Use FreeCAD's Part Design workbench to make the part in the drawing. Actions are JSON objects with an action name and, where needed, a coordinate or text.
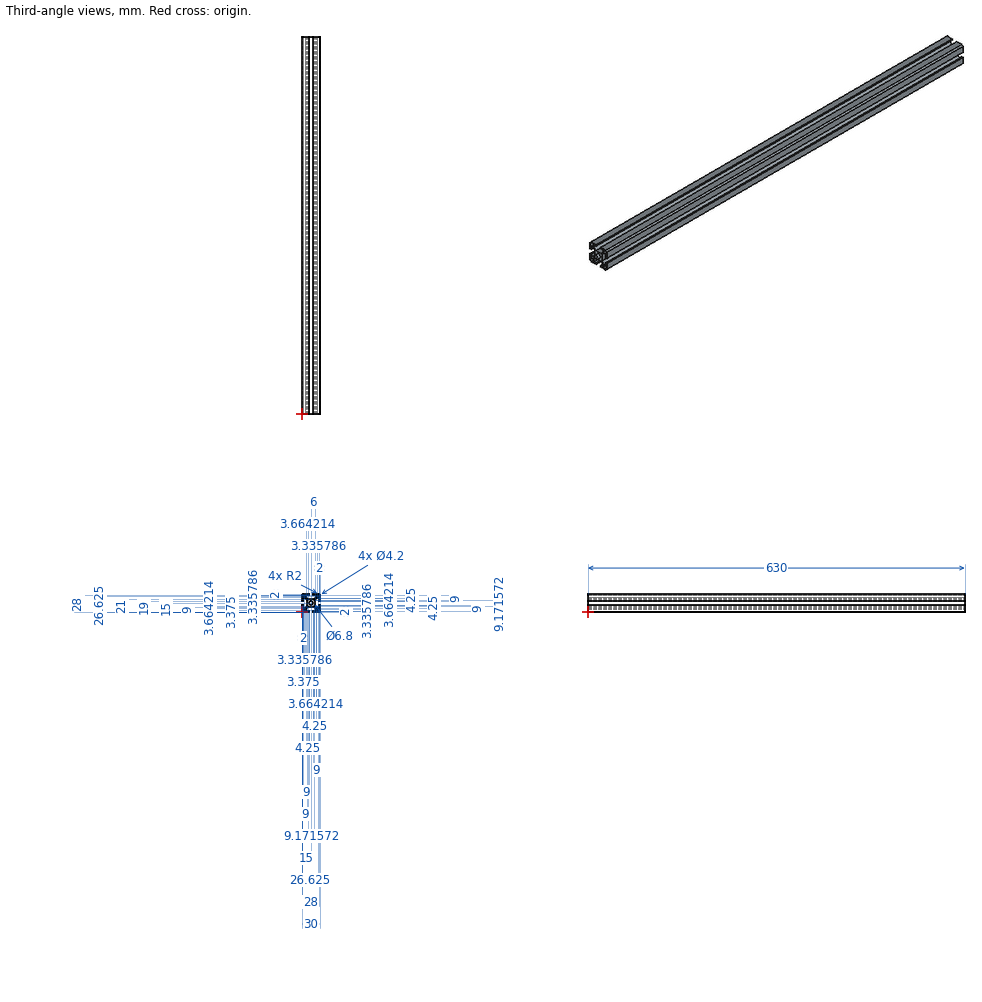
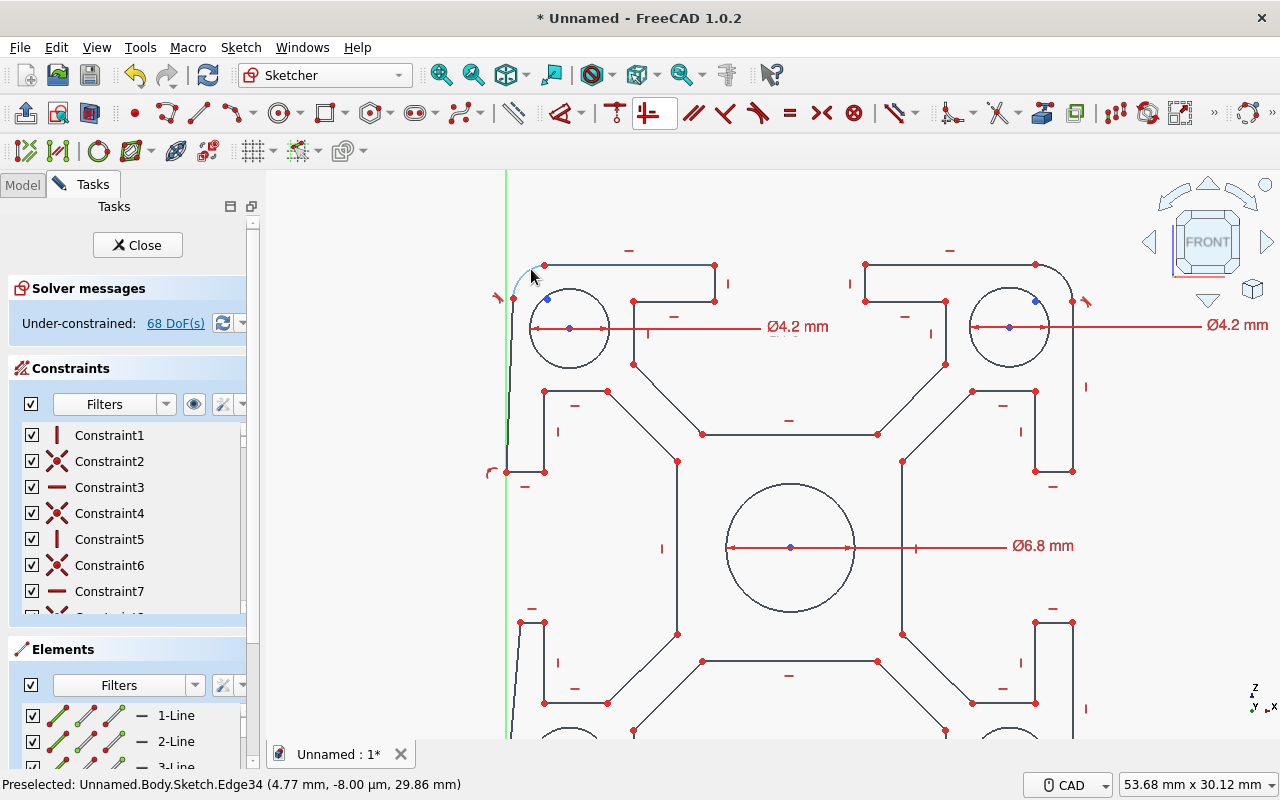
{"action": "left_click", "coordinate": [531, 270]}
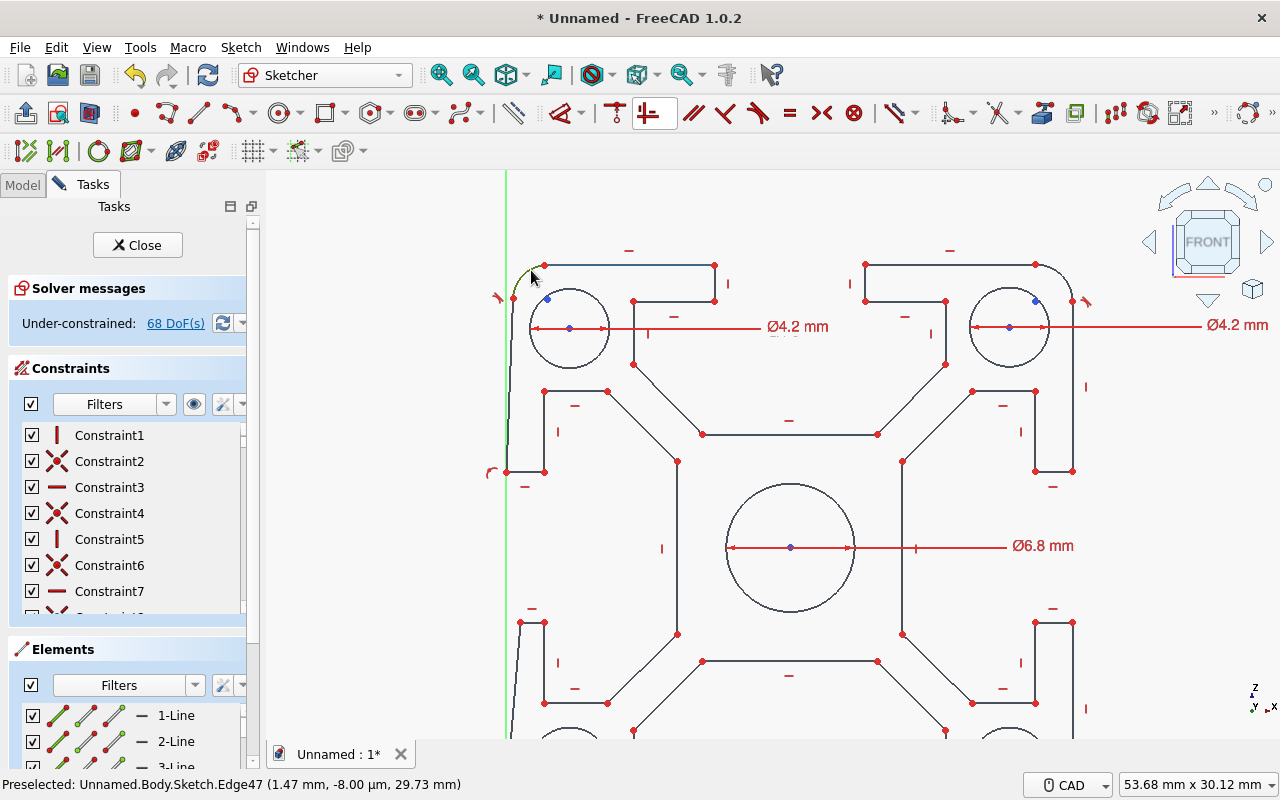
{"action": "left_click", "coordinate": [758, 114]}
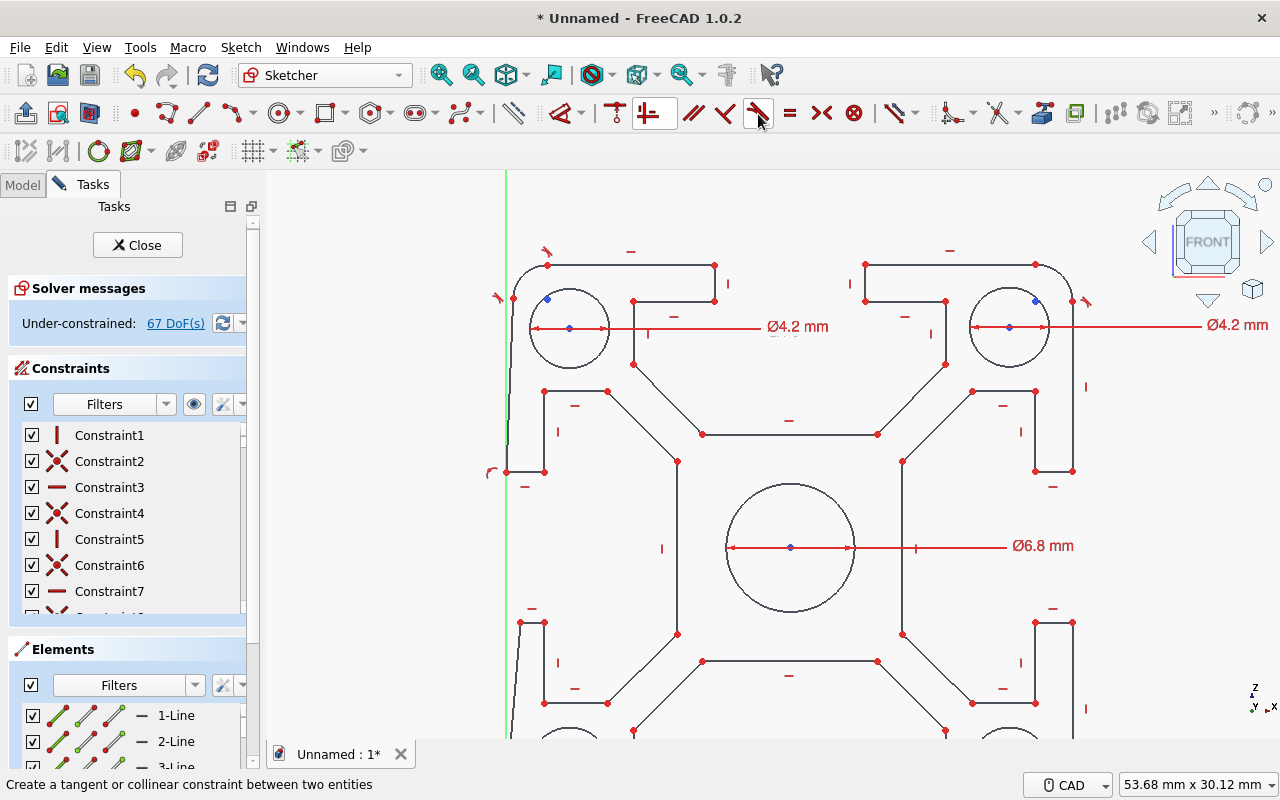
{"action": "left_click", "coordinate": [916, 265]}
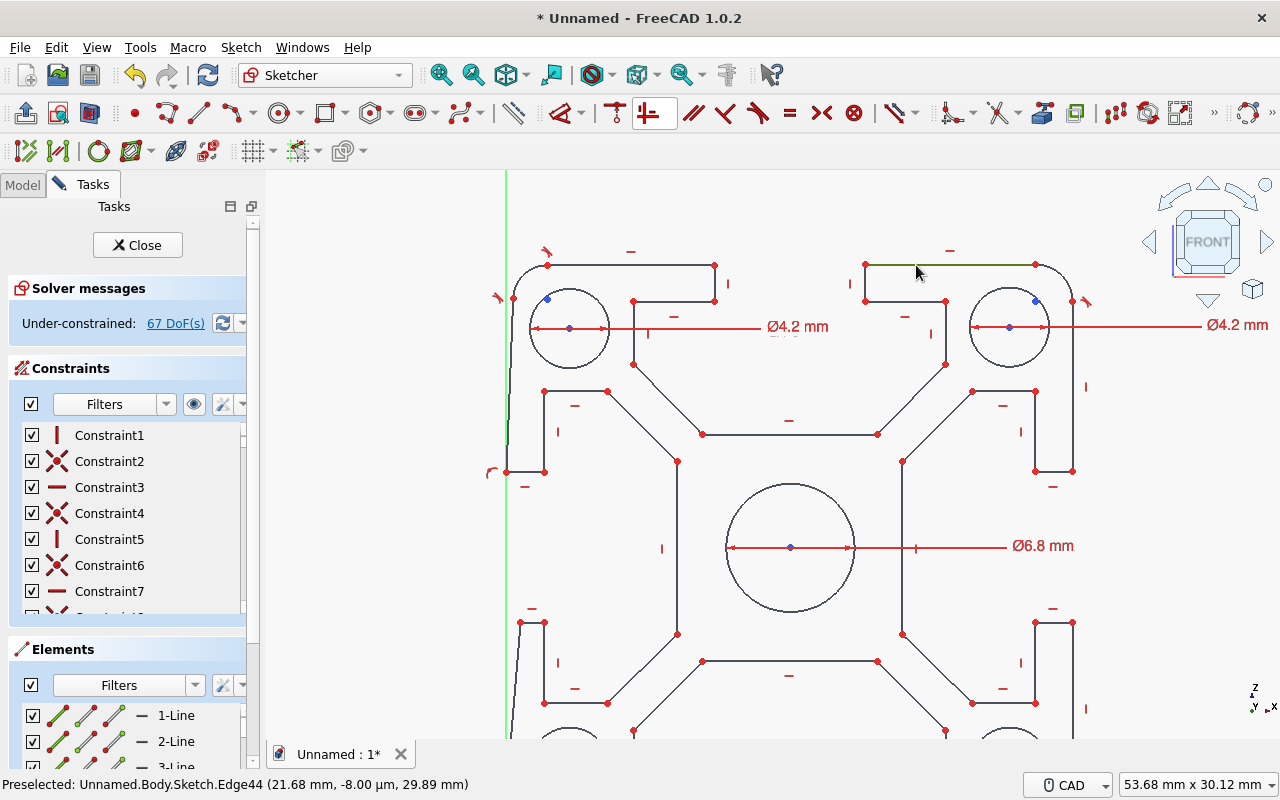
{"action": "left_click", "coordinate": [1069, 285]}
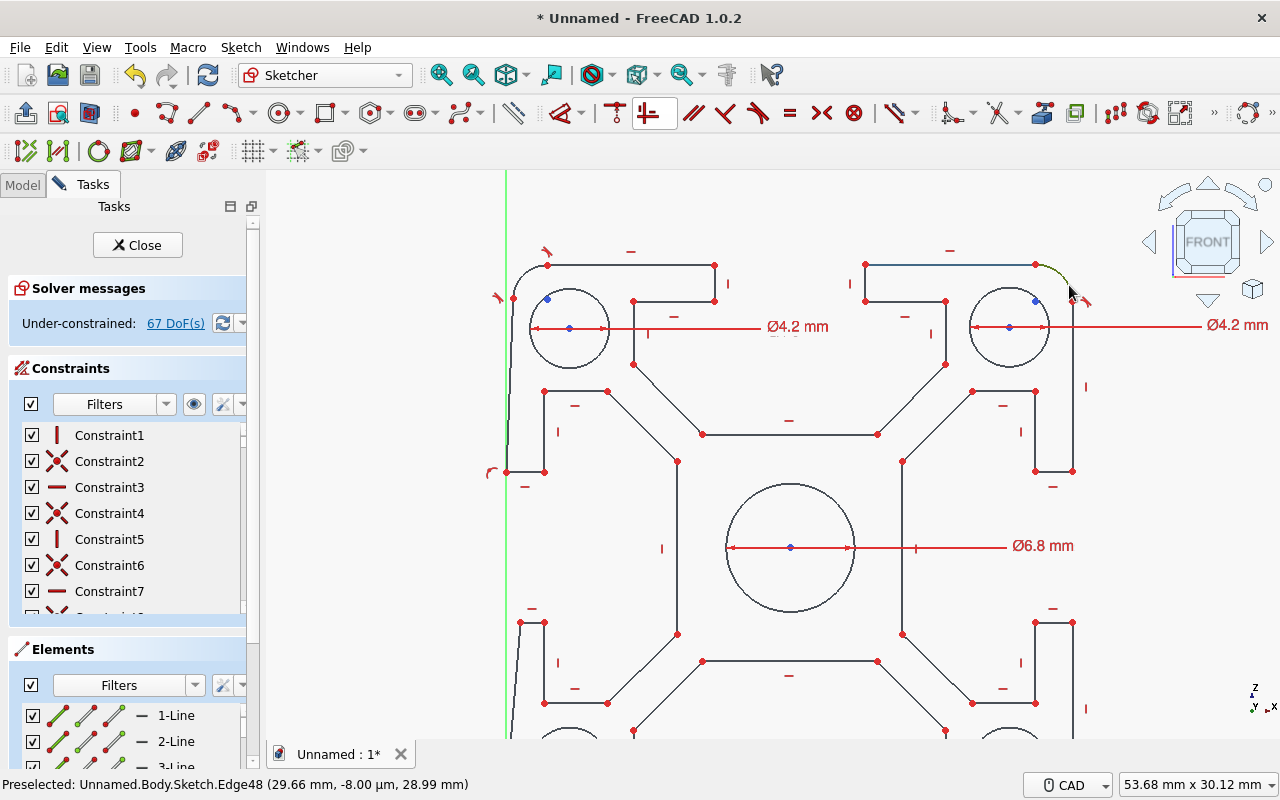
{"action": "key", "text": "t"}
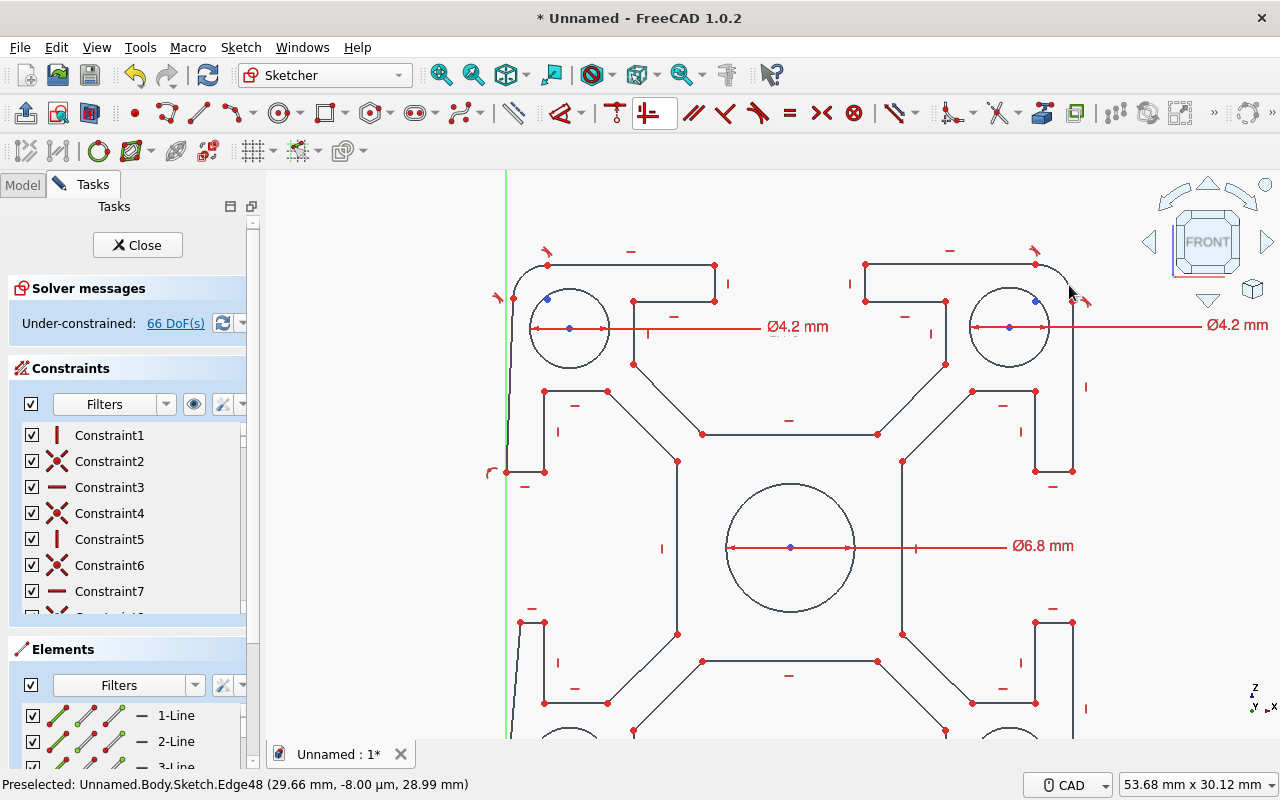
{"action": "scroll", "coordinate": [531, 269], "scroll_direction": "down", "scroll_amount": 2}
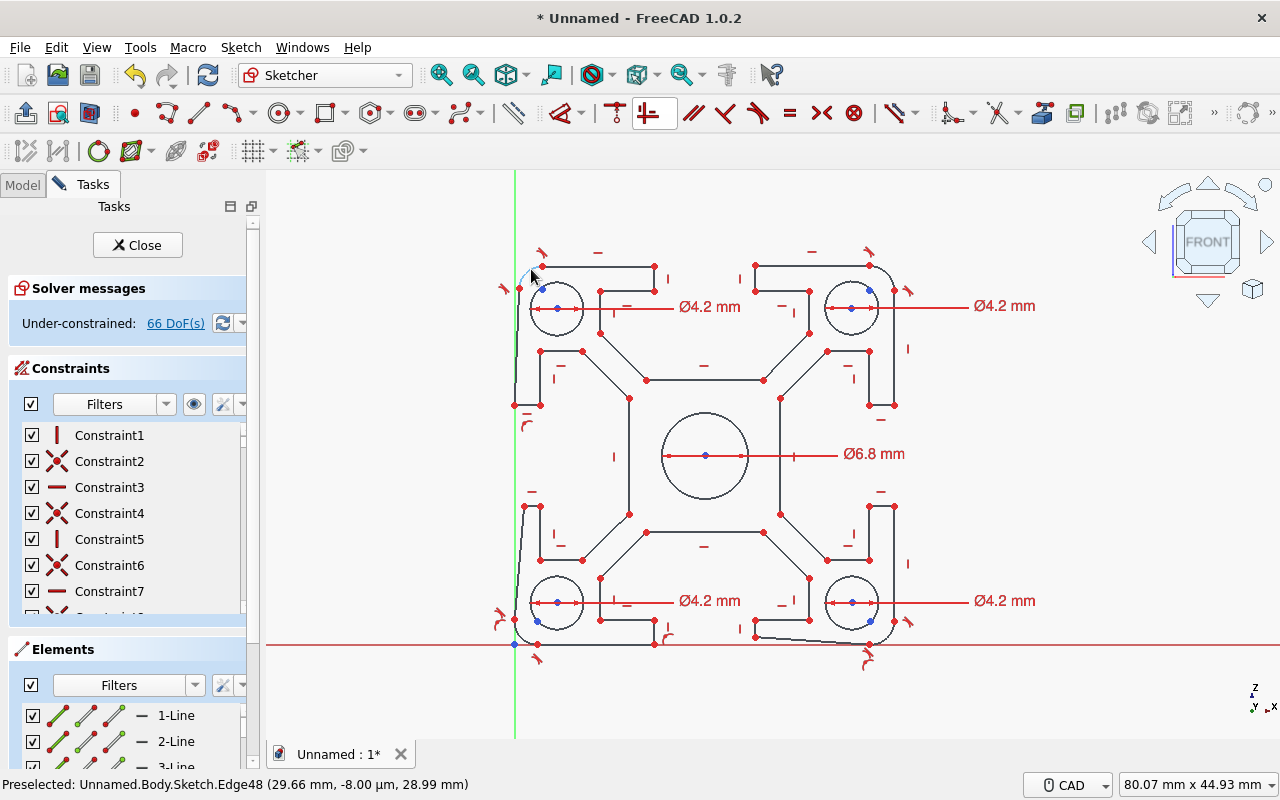
{"action": "left_click", "coordinate": [835, 642]}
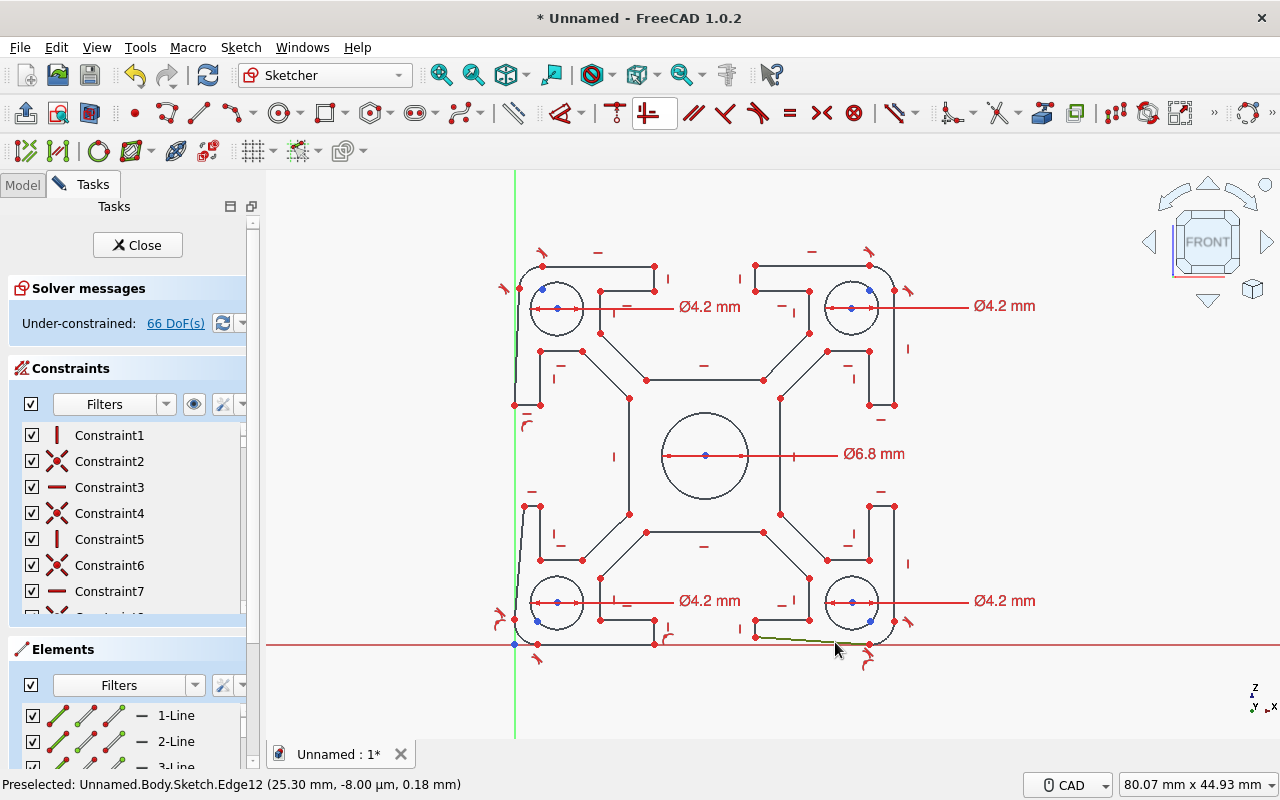
{"action": "key", "text": "h"}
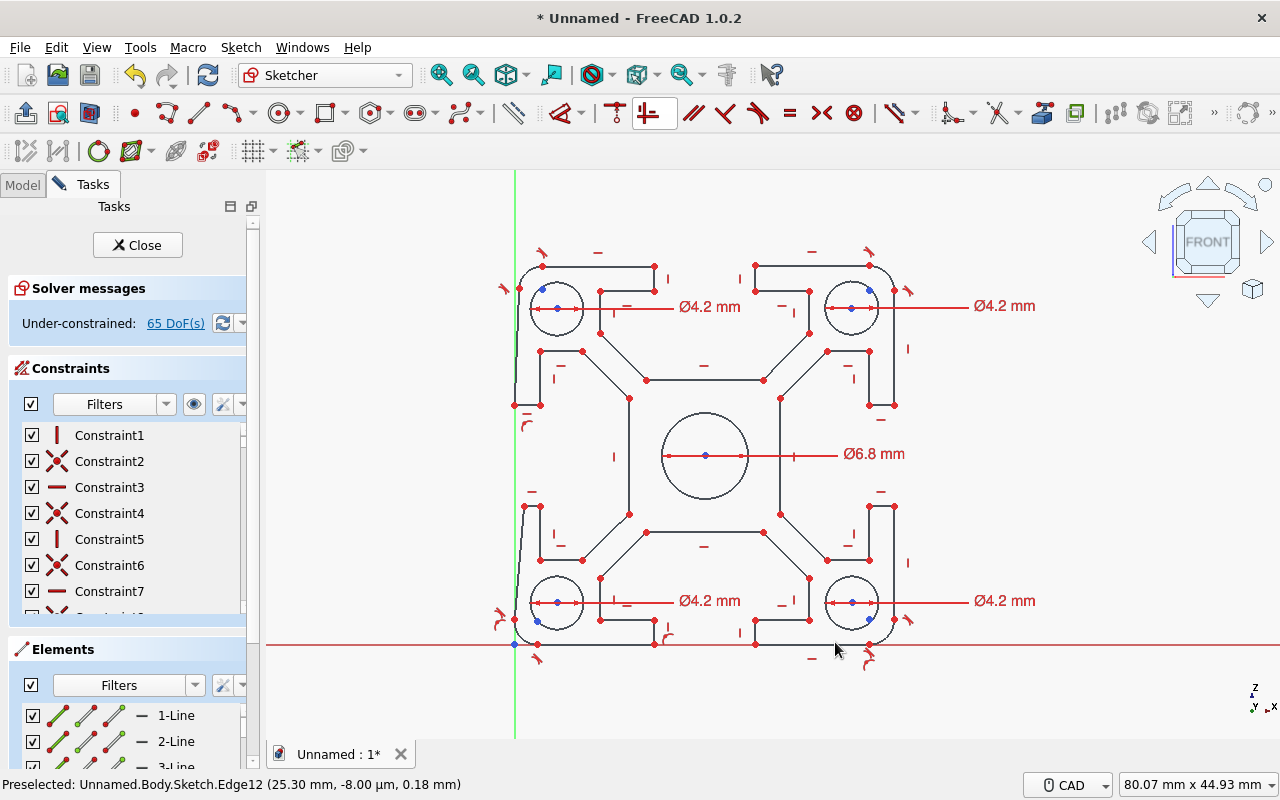
{"action": "left_click", "coordinate": [619, 645]}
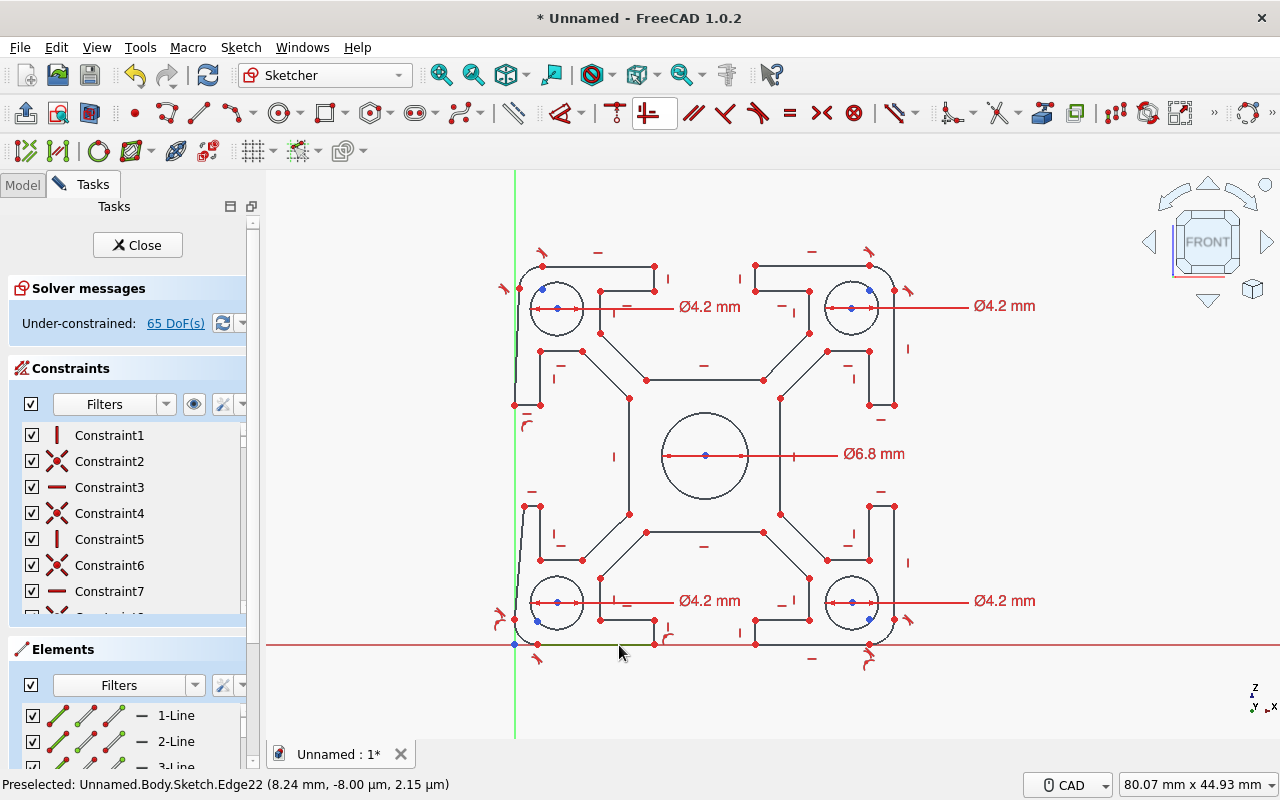
{"action": "left_click", "coordinate": [672, 114]}